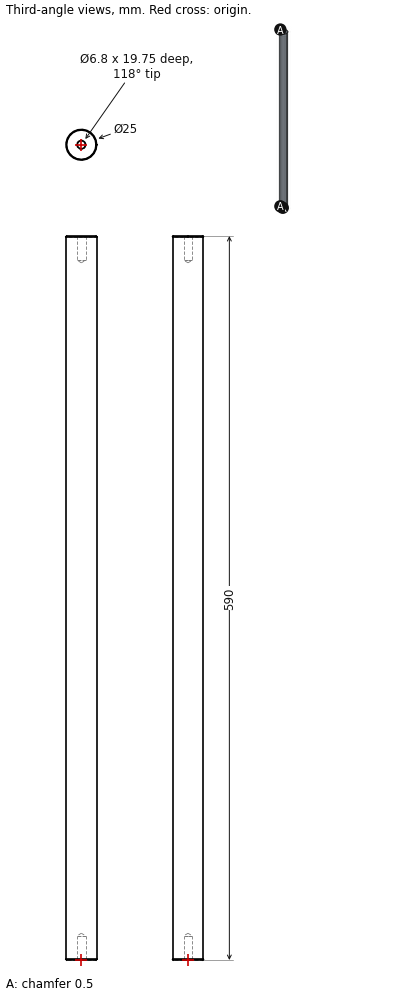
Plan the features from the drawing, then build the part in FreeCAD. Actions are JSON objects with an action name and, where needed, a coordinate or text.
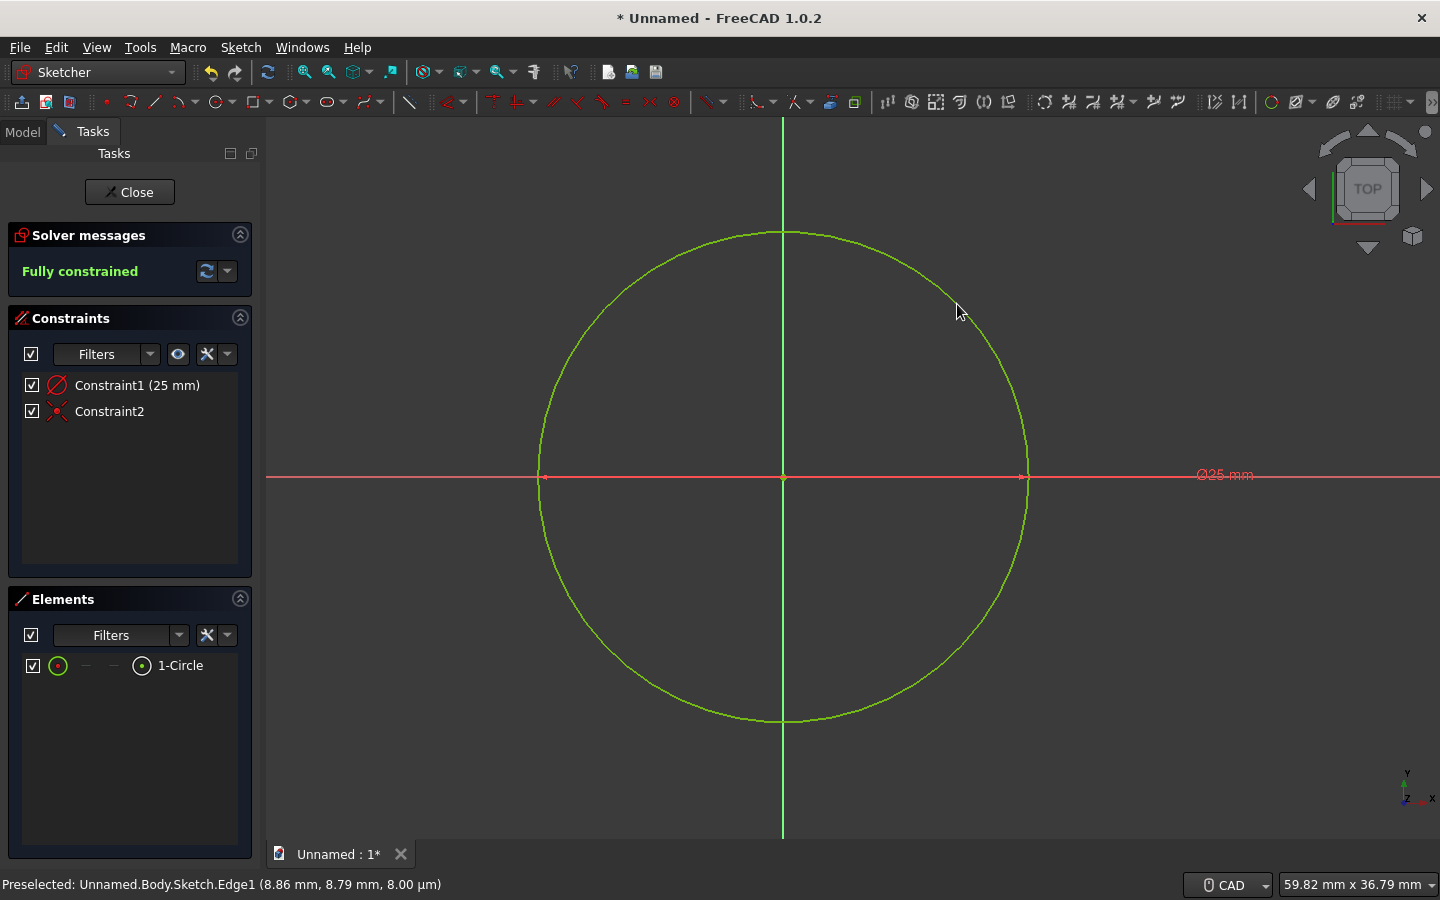
{"action": "left_click", "coordinate": [130, 192]}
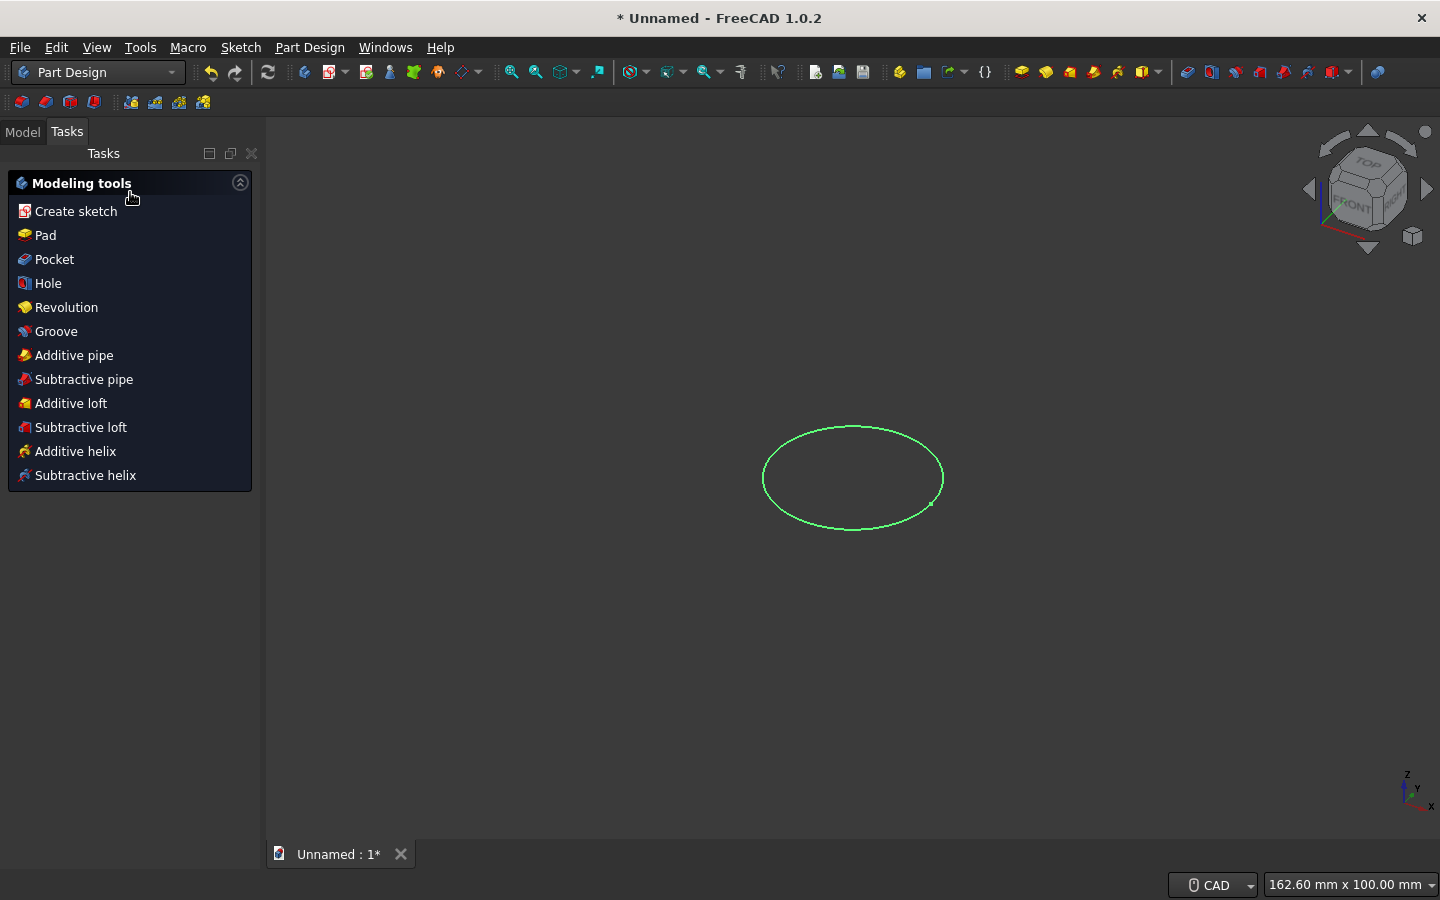
{"action": "left_click", "coordinate": [1022, 72]}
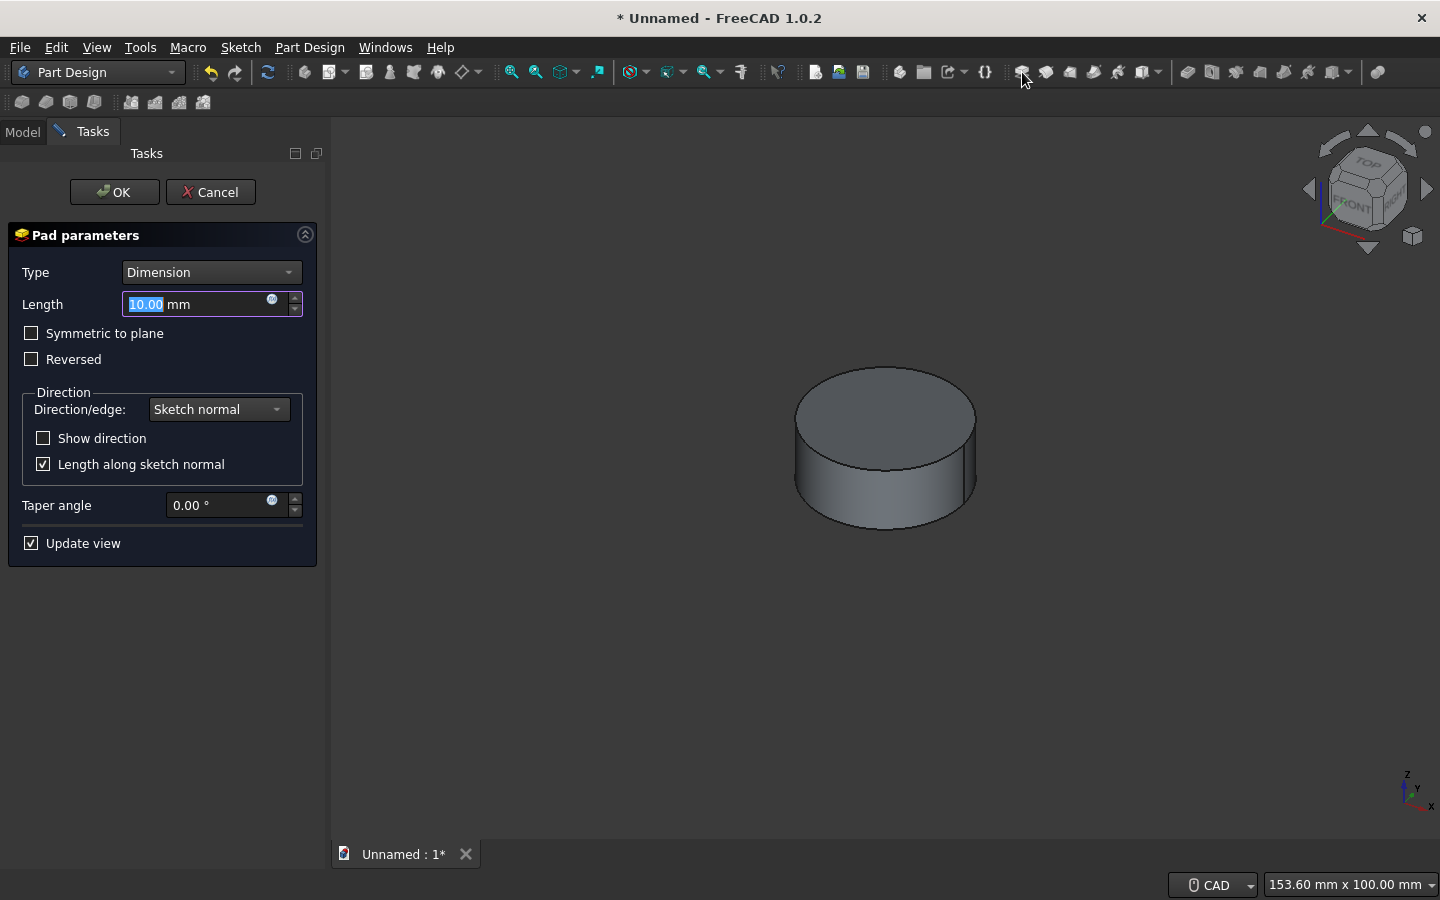
{"action": "type", "text": "590"}
{"action": "key", "text": "Tab"}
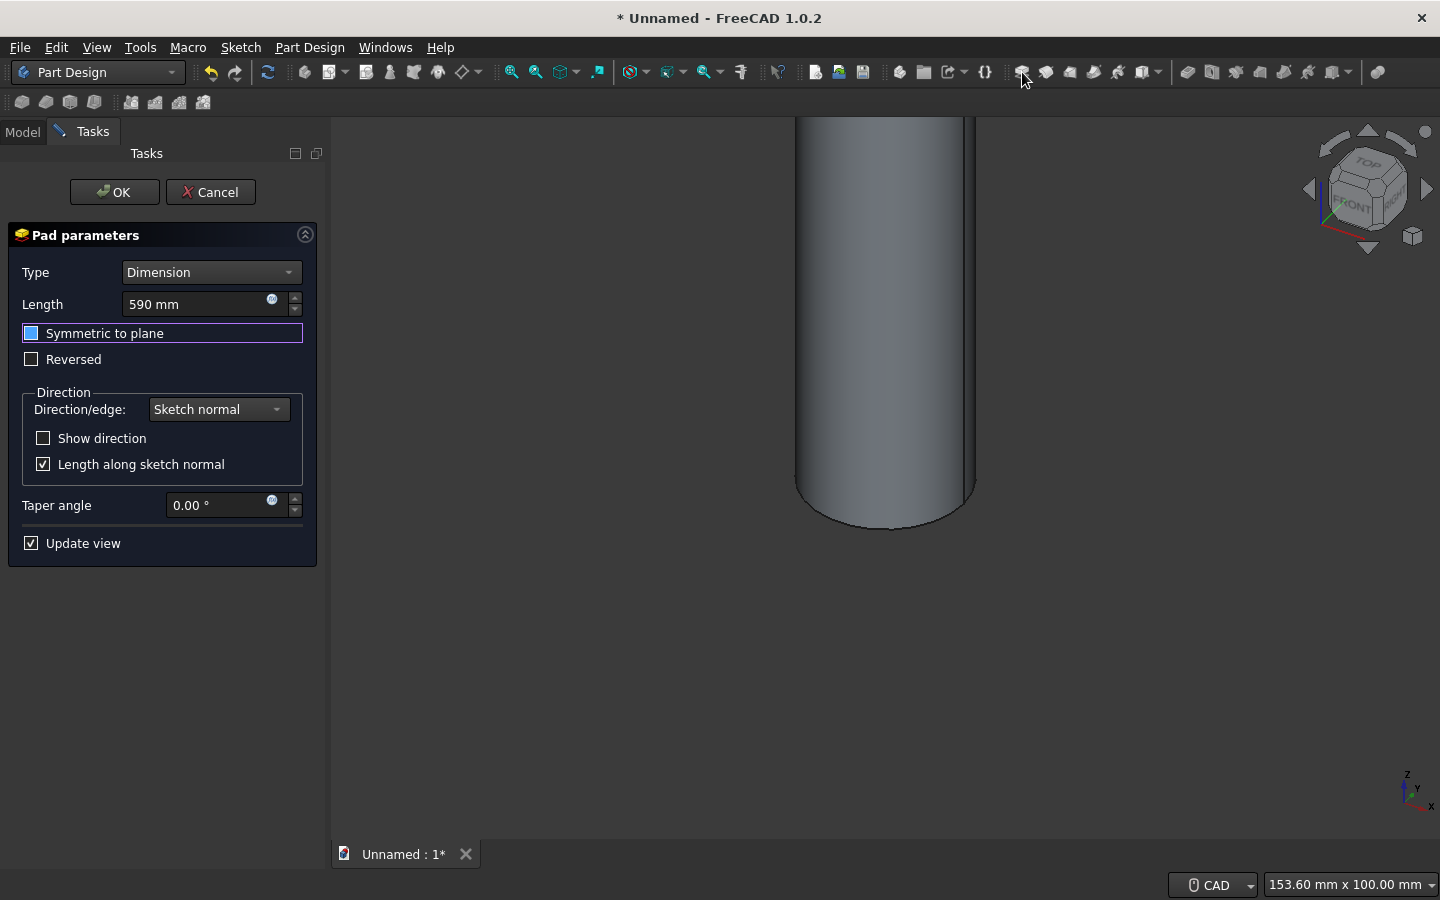
{"action": "left_click", "coordinate": [115, 192]}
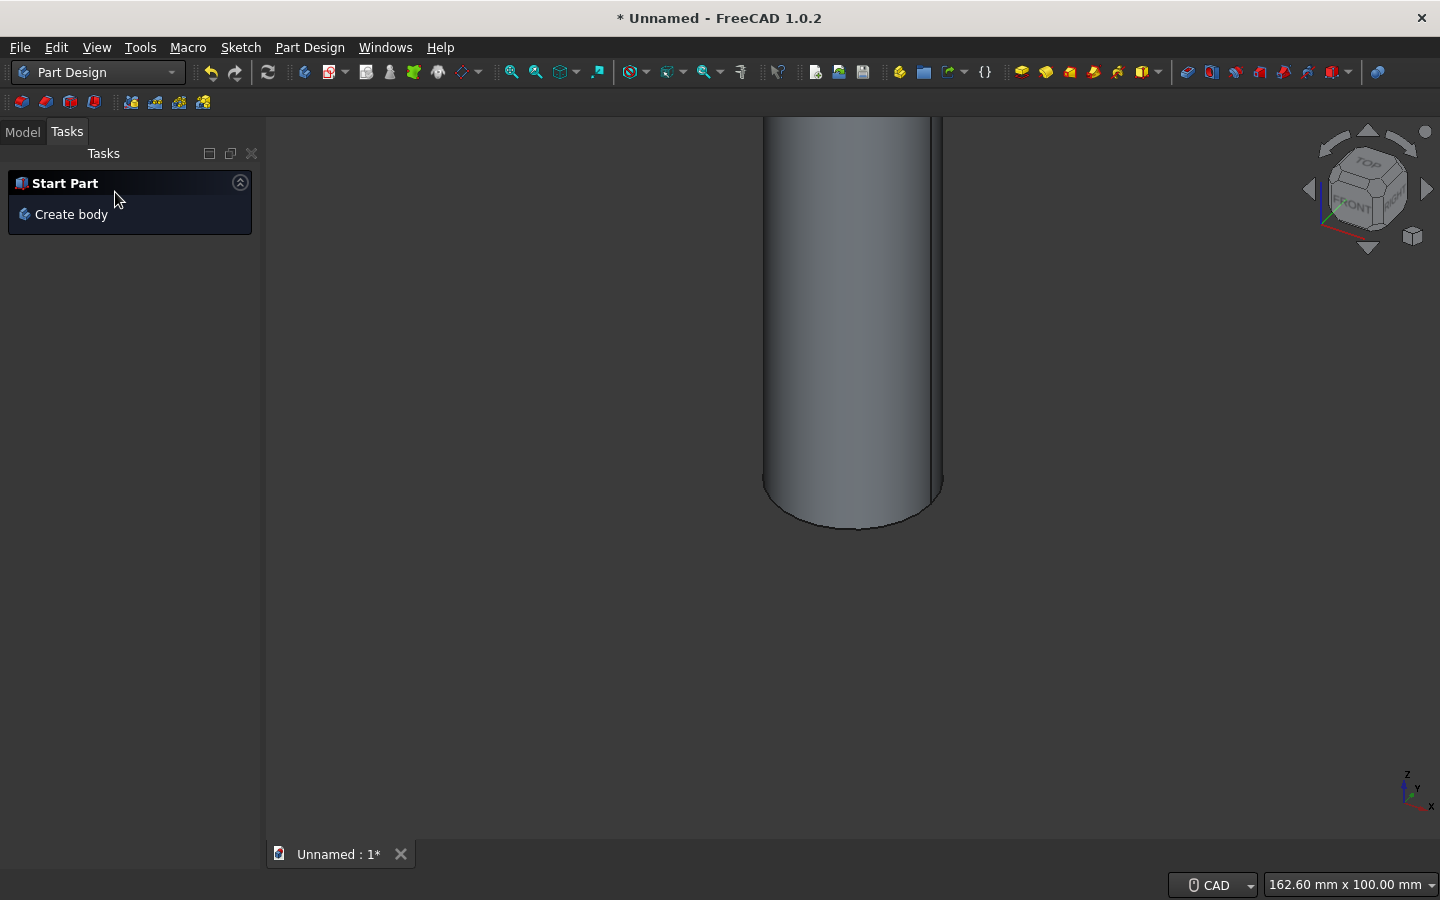
{"action": "key", "text": "v f"}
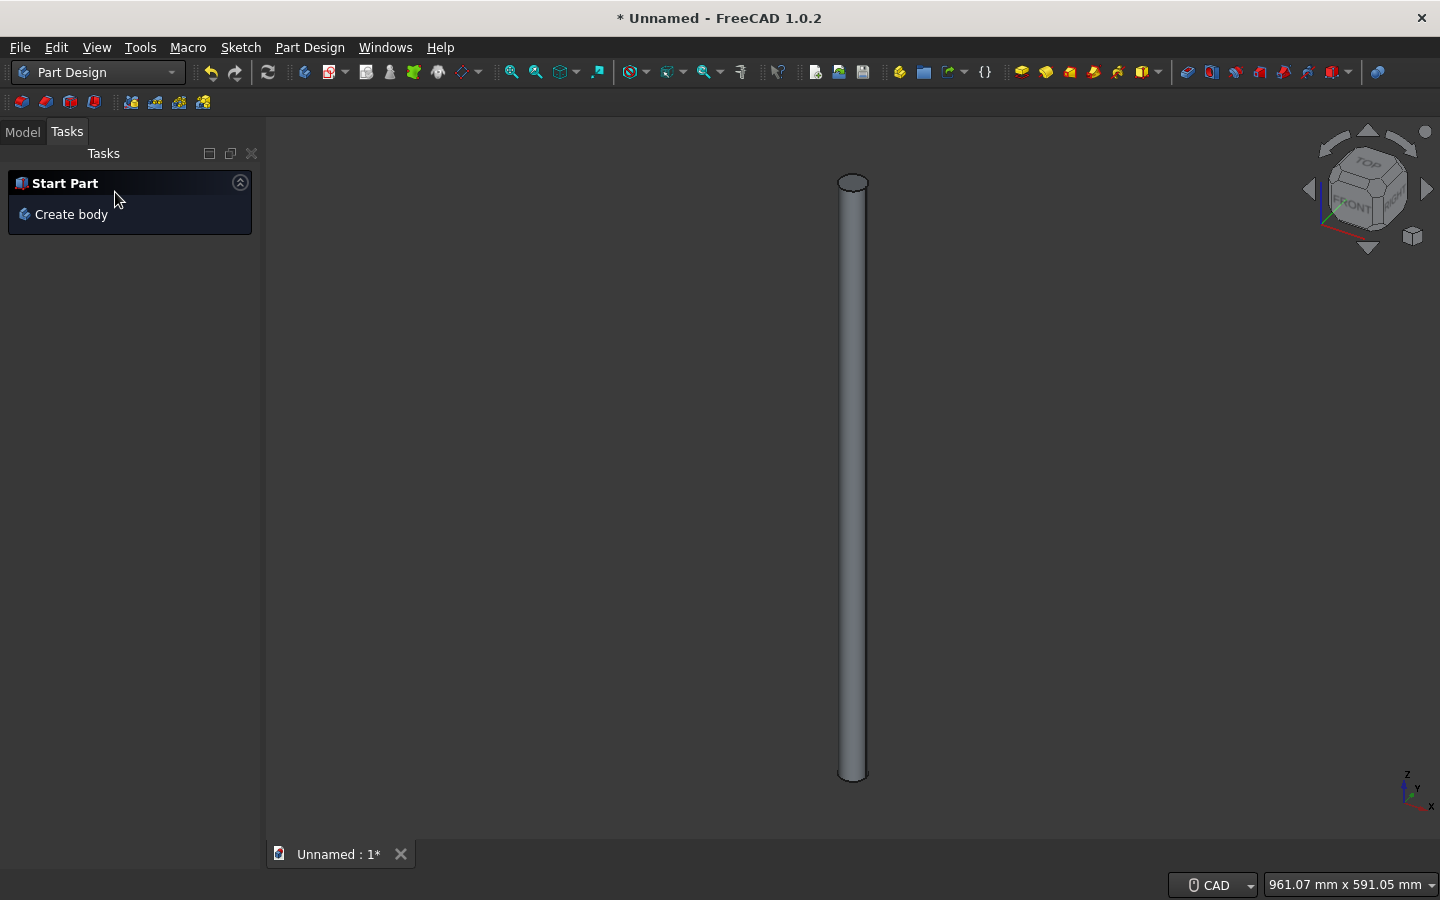
{"action": "left_click", "coordinate": [853, 182]}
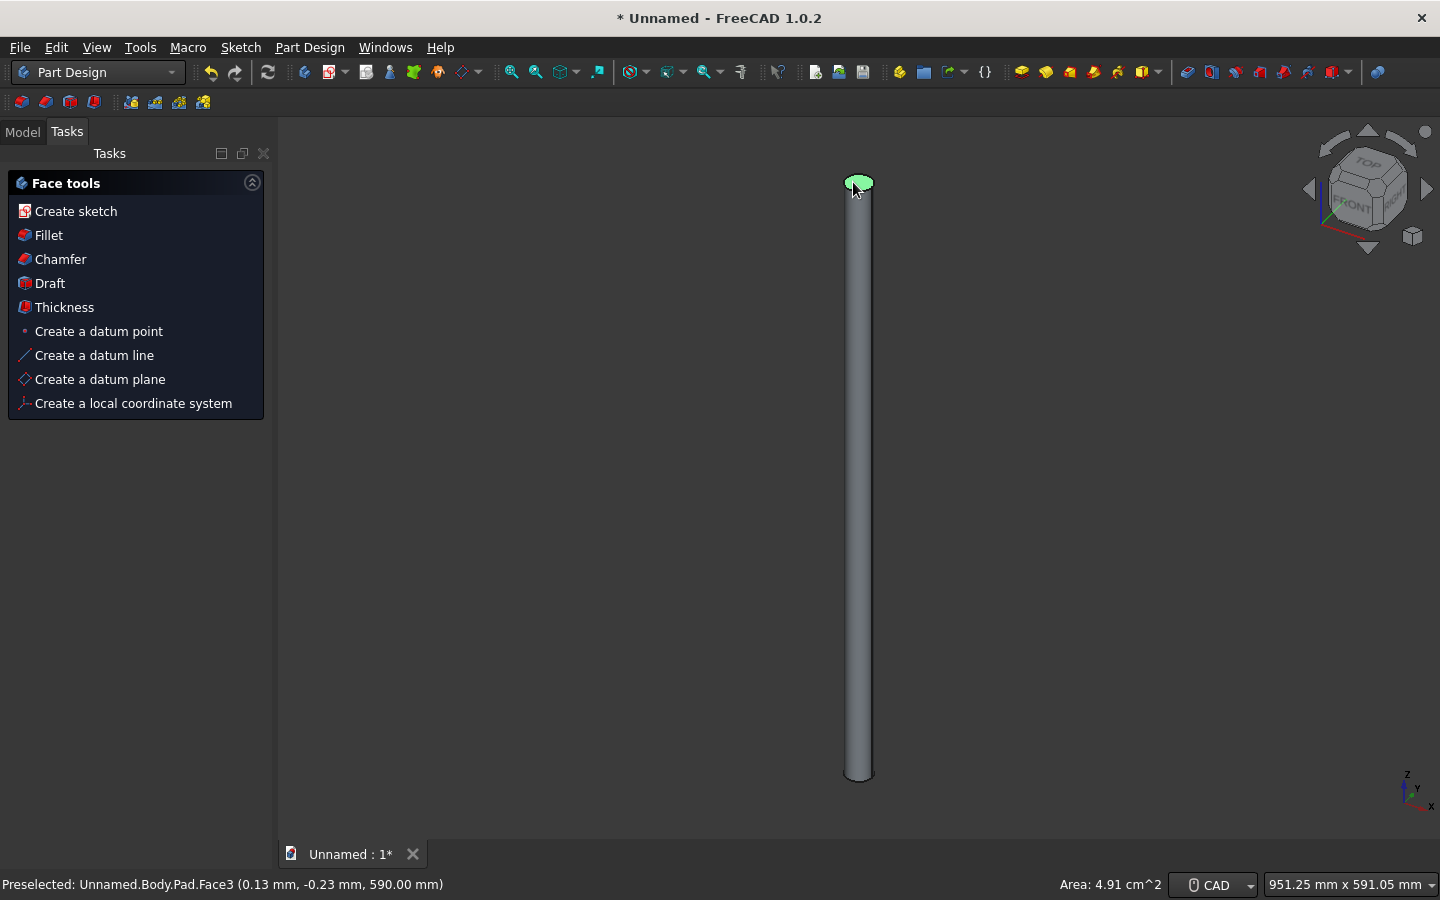
{"action": "left_click", "coordinate": [330, 72]}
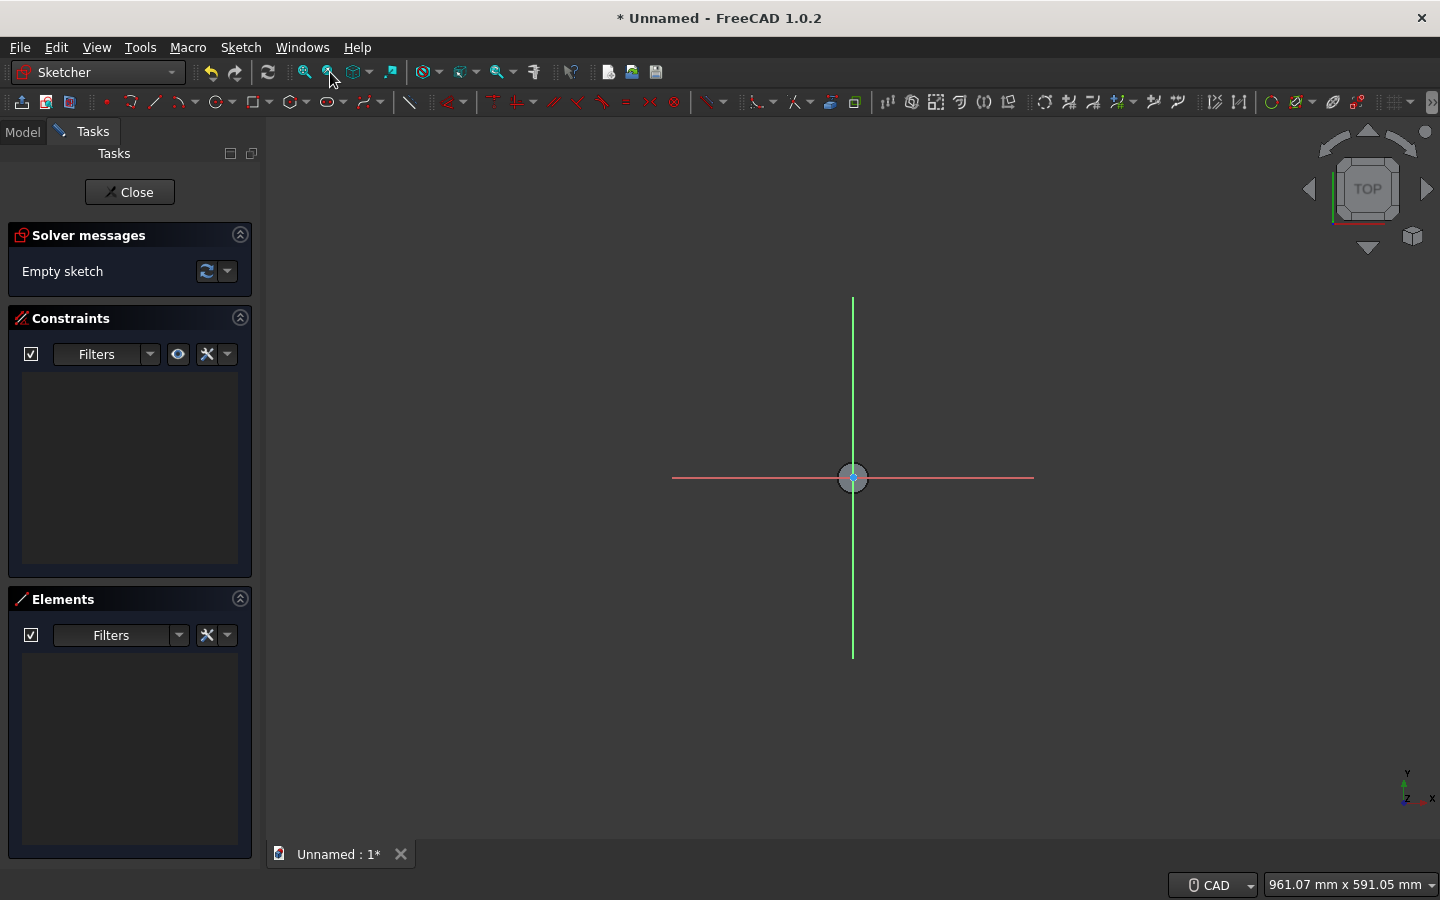
{"action": "scroll", "coordinate": [857, 478], "scroll_direction": "up", "scroll_amount": 15}